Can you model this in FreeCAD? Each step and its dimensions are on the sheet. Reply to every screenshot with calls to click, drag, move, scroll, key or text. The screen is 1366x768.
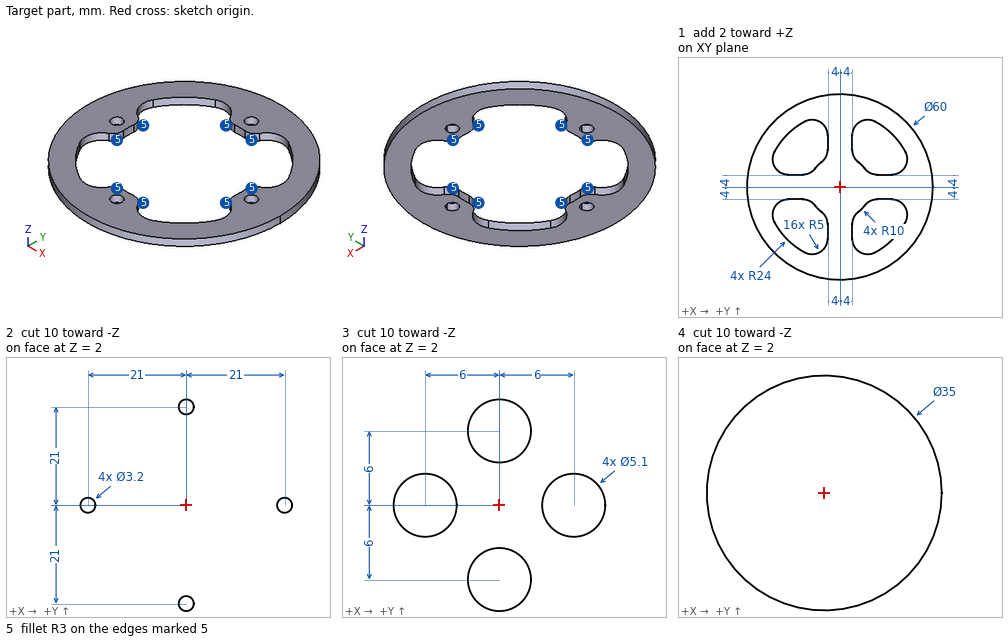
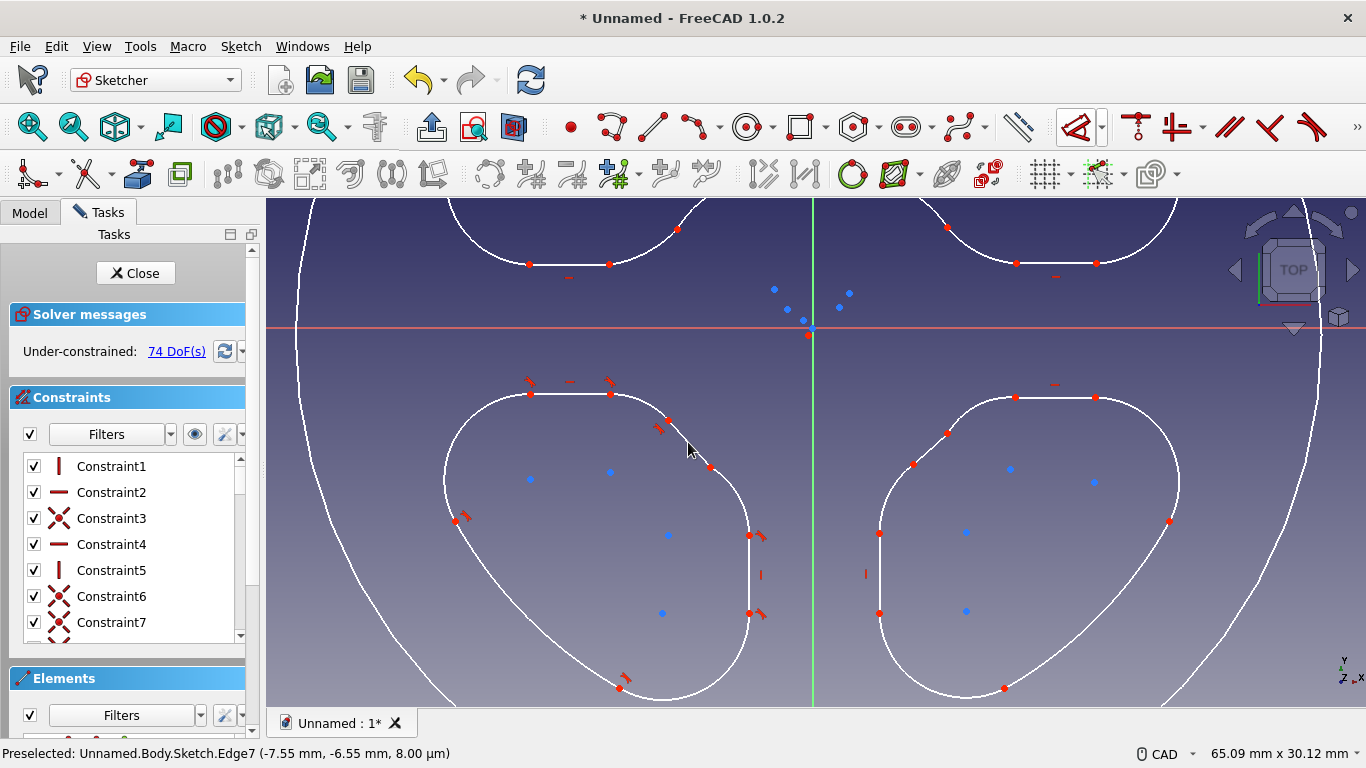
click(681, 435)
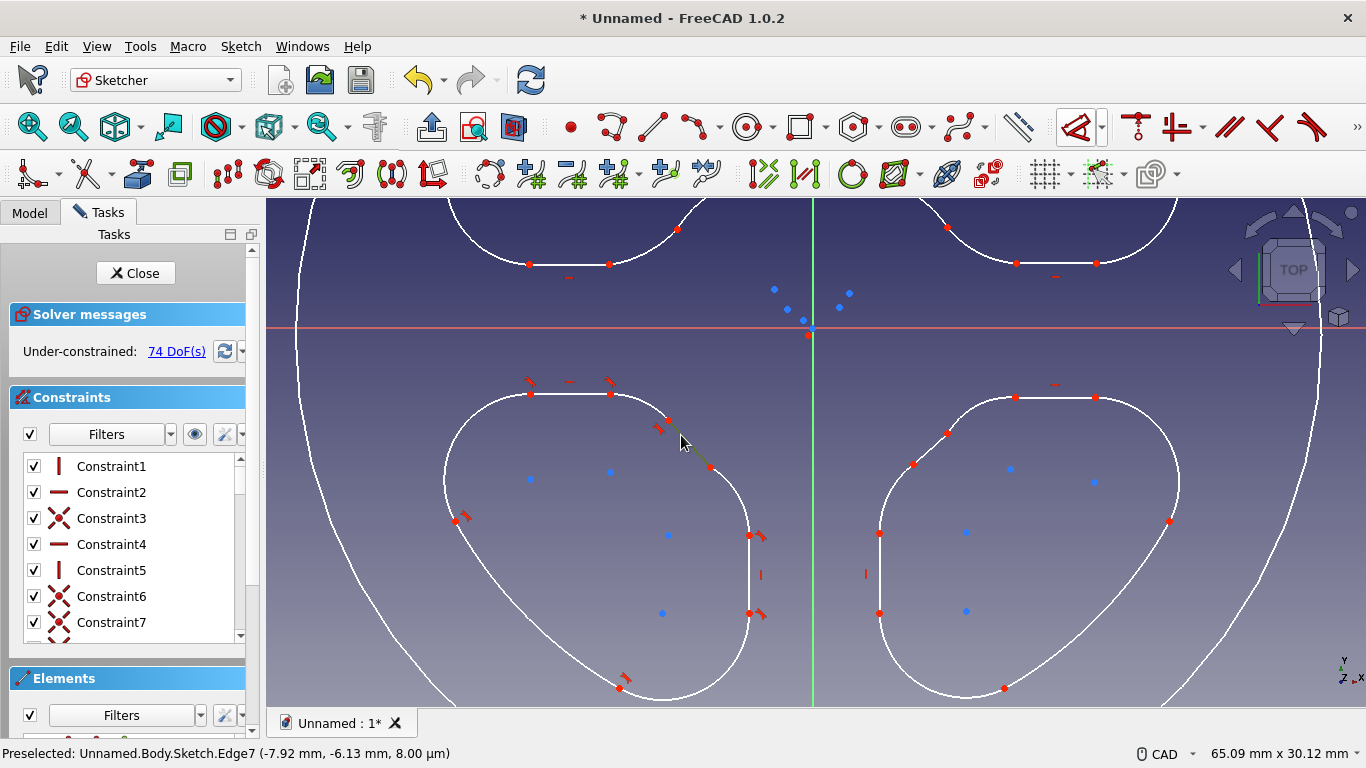
click(745, 512)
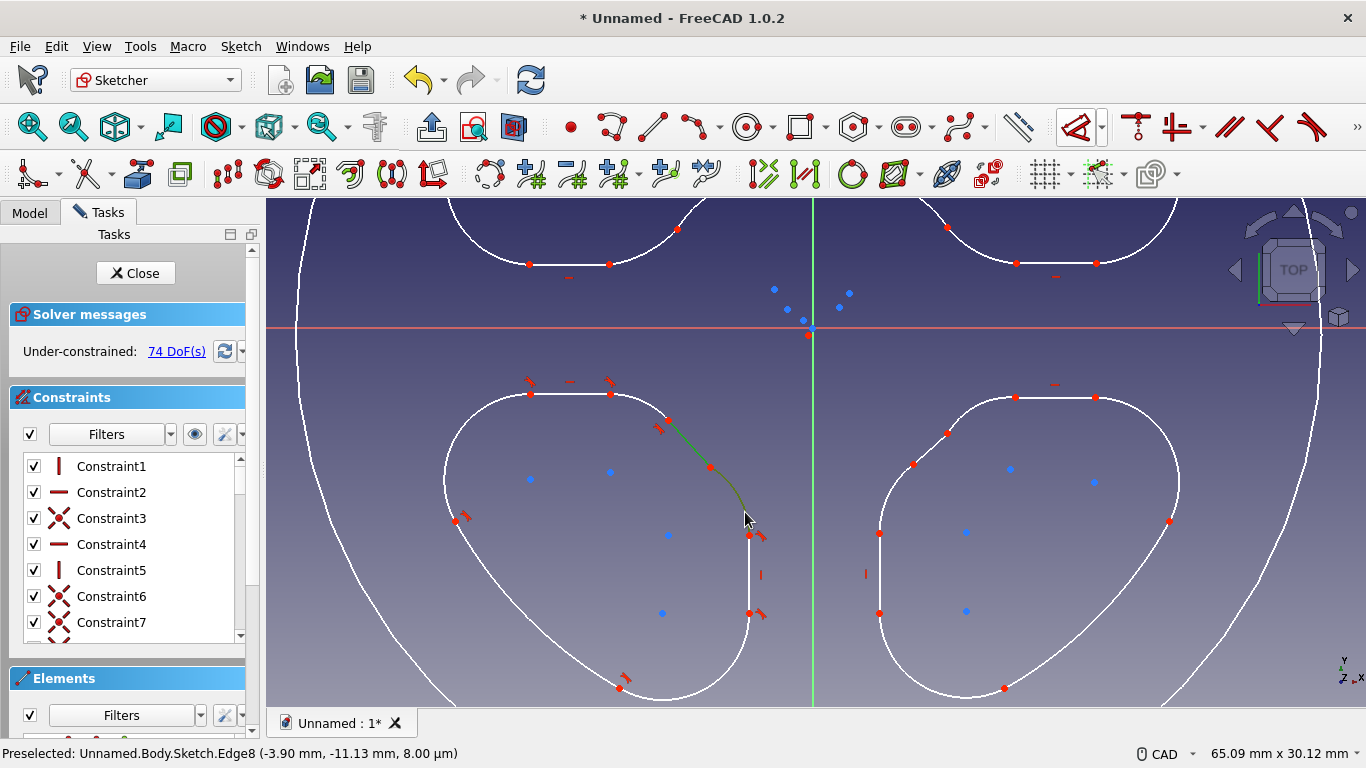
key(t)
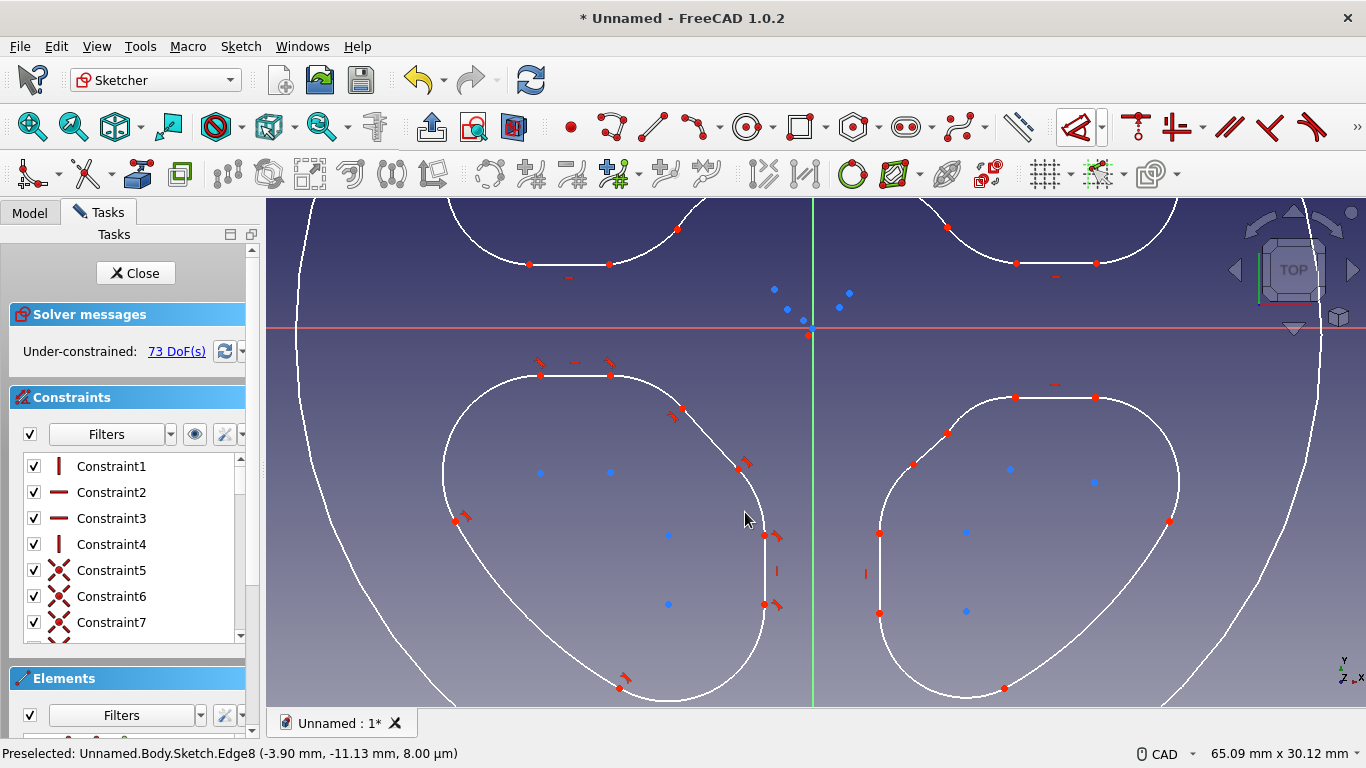
click(1040, 398)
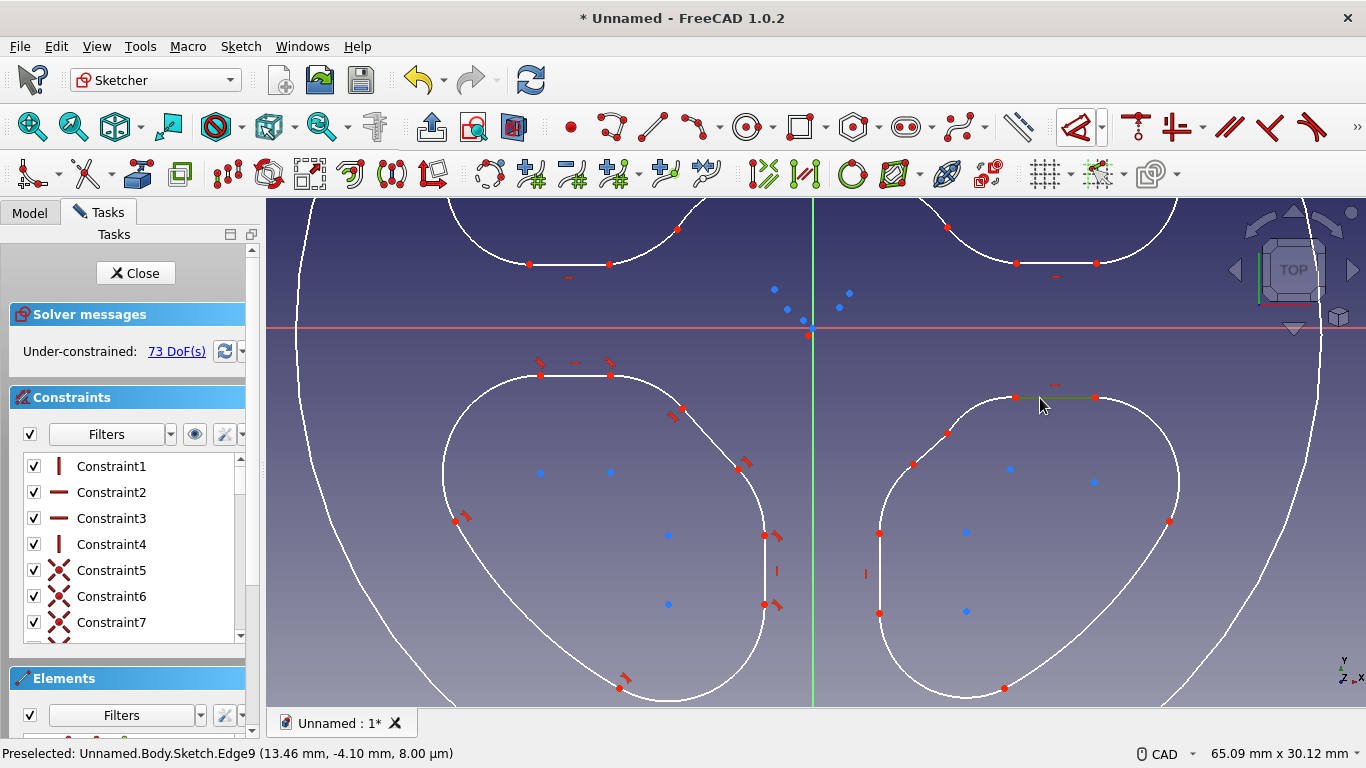
click(1178, 471)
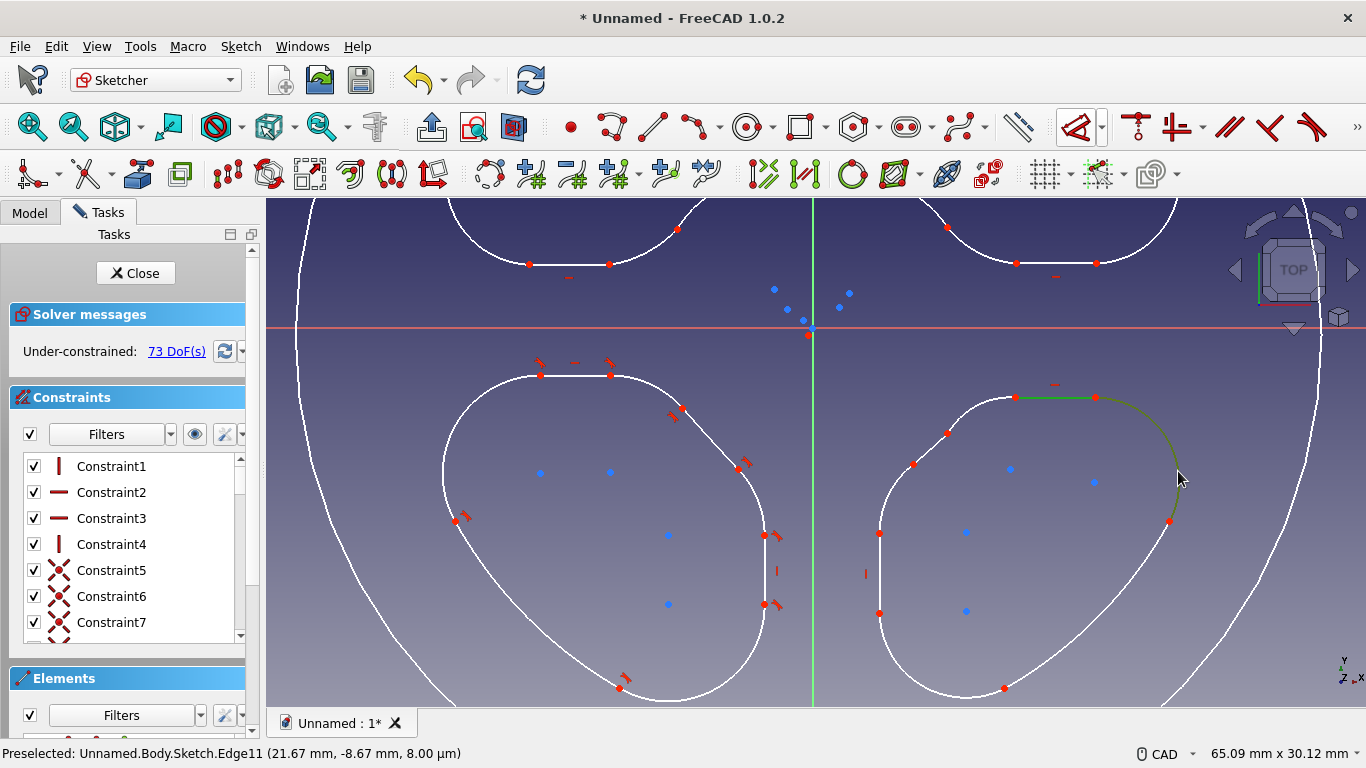
key(t)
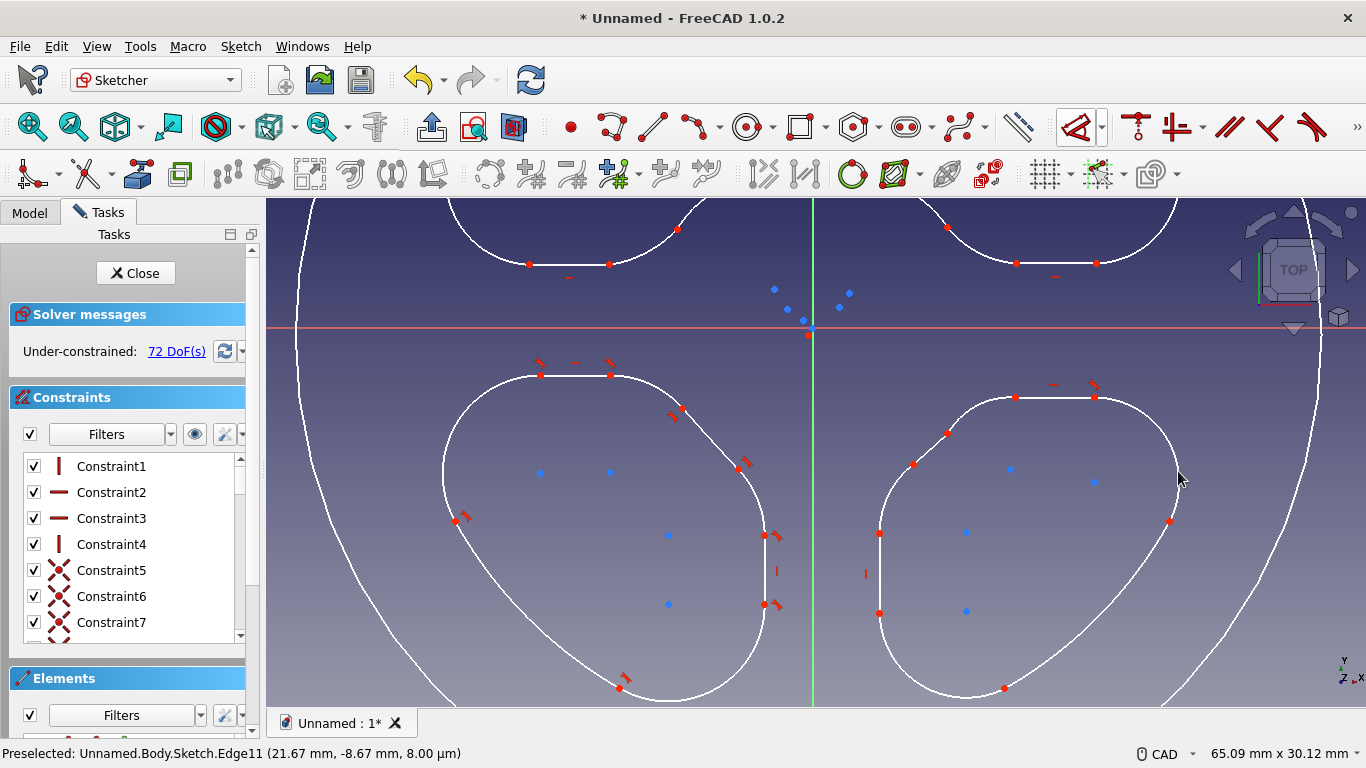
click(1039, 398)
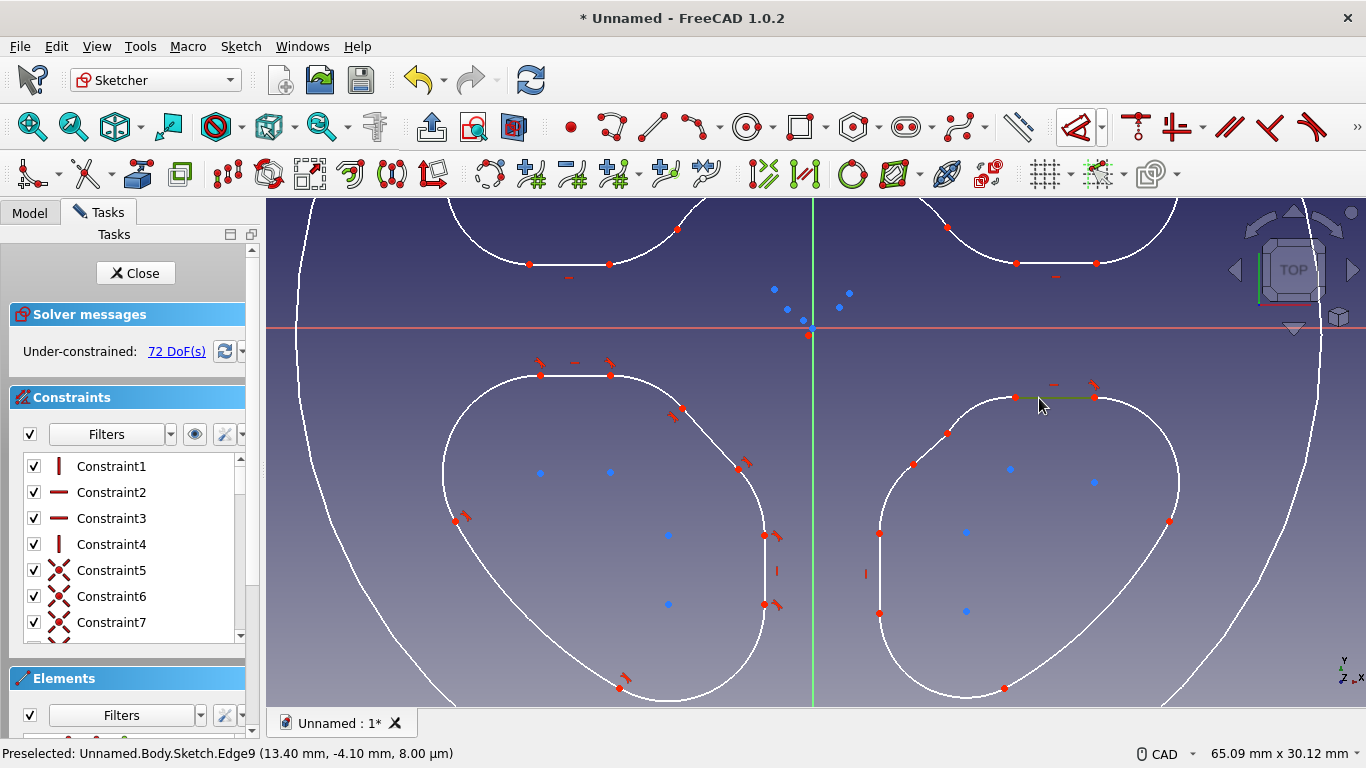
click(992, 400)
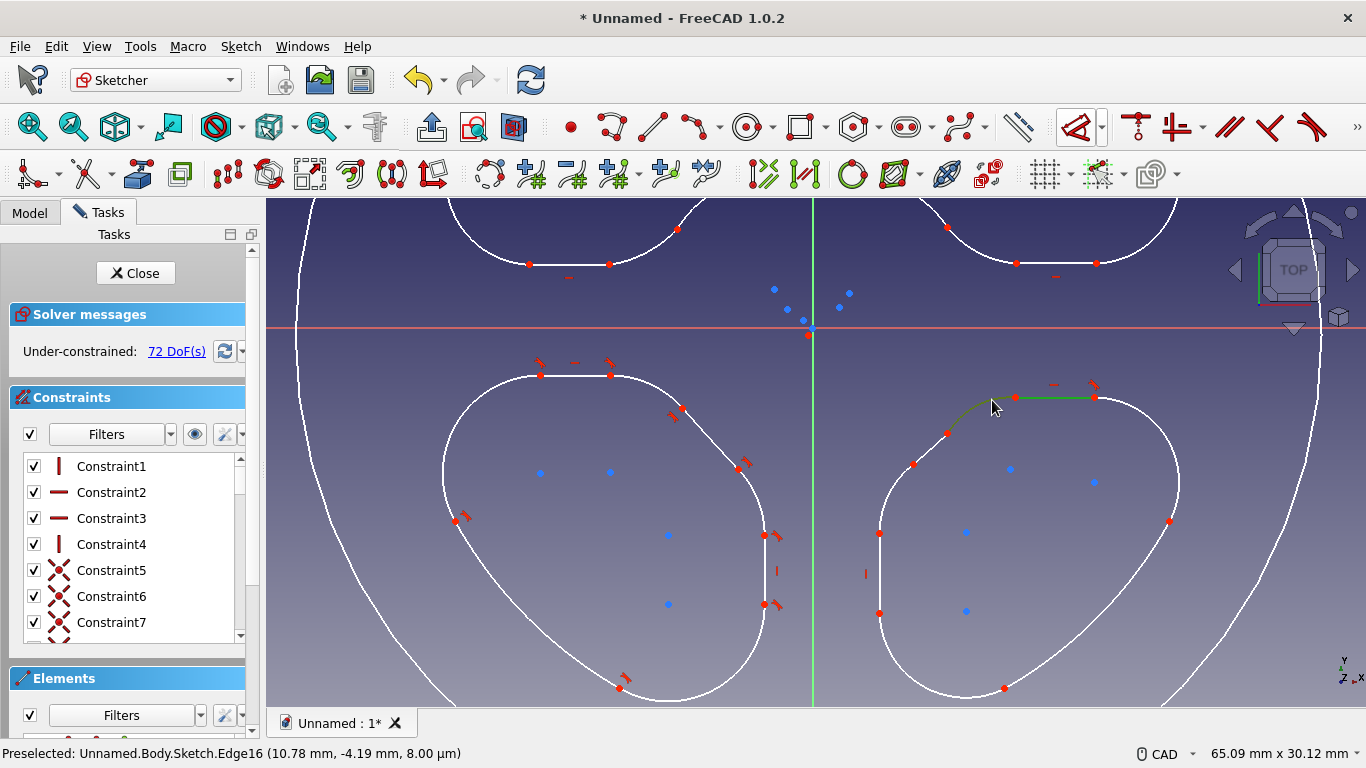
key(t)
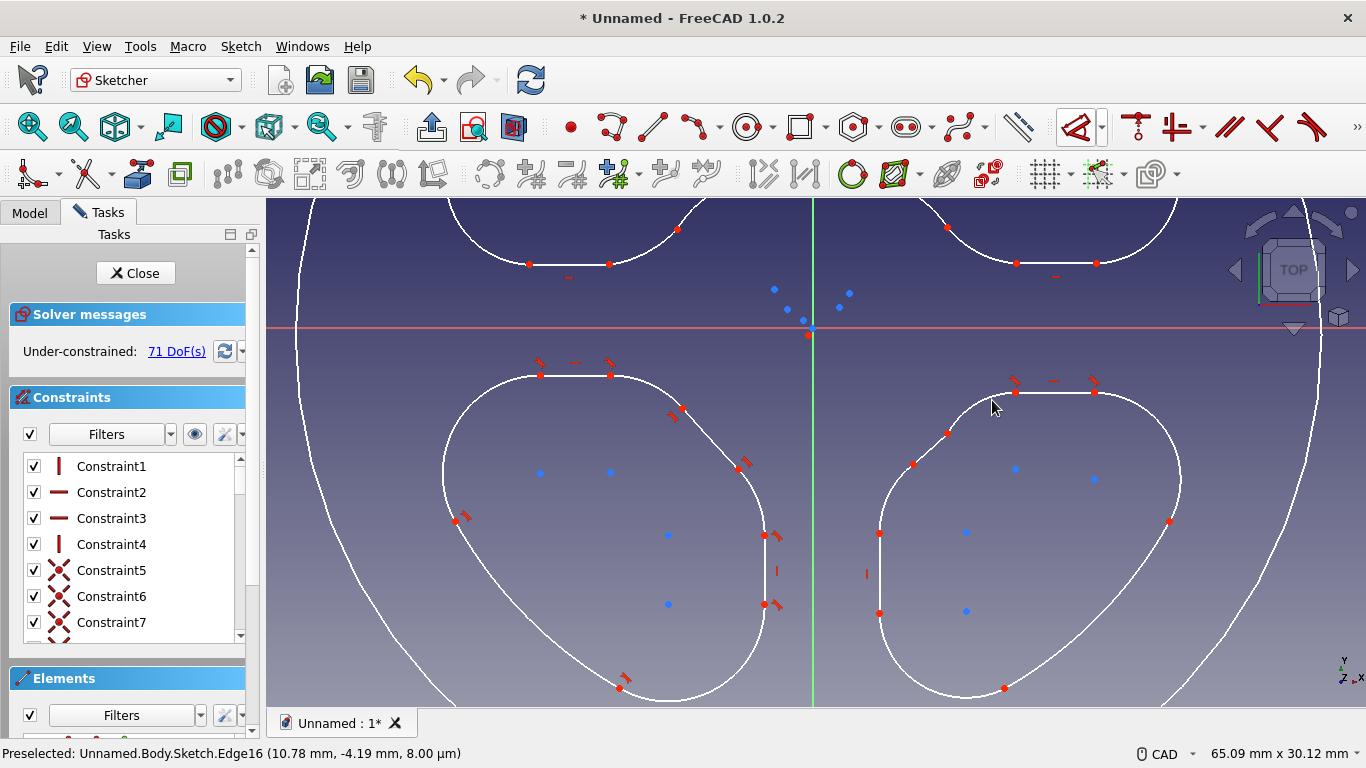
click(880, 589)